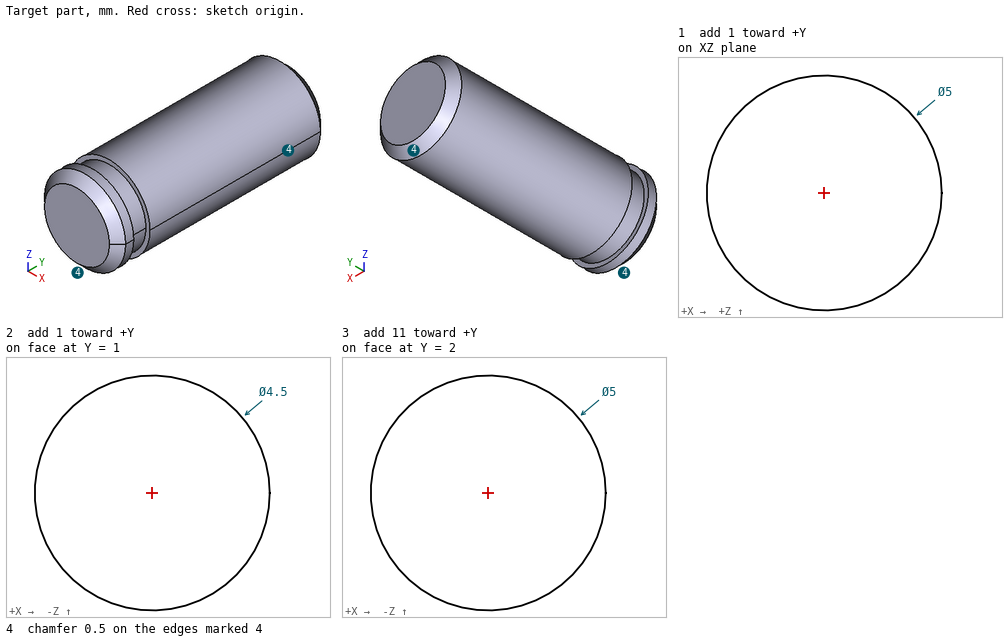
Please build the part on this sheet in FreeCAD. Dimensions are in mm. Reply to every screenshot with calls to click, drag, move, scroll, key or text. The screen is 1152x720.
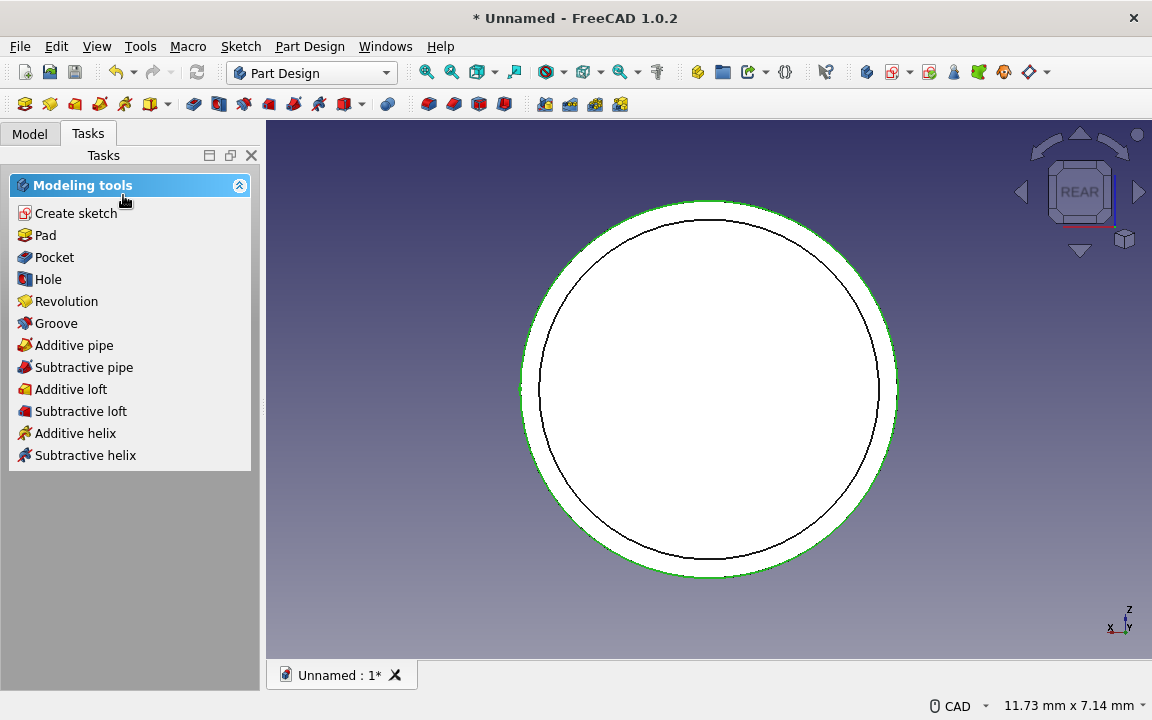
click(25, 104)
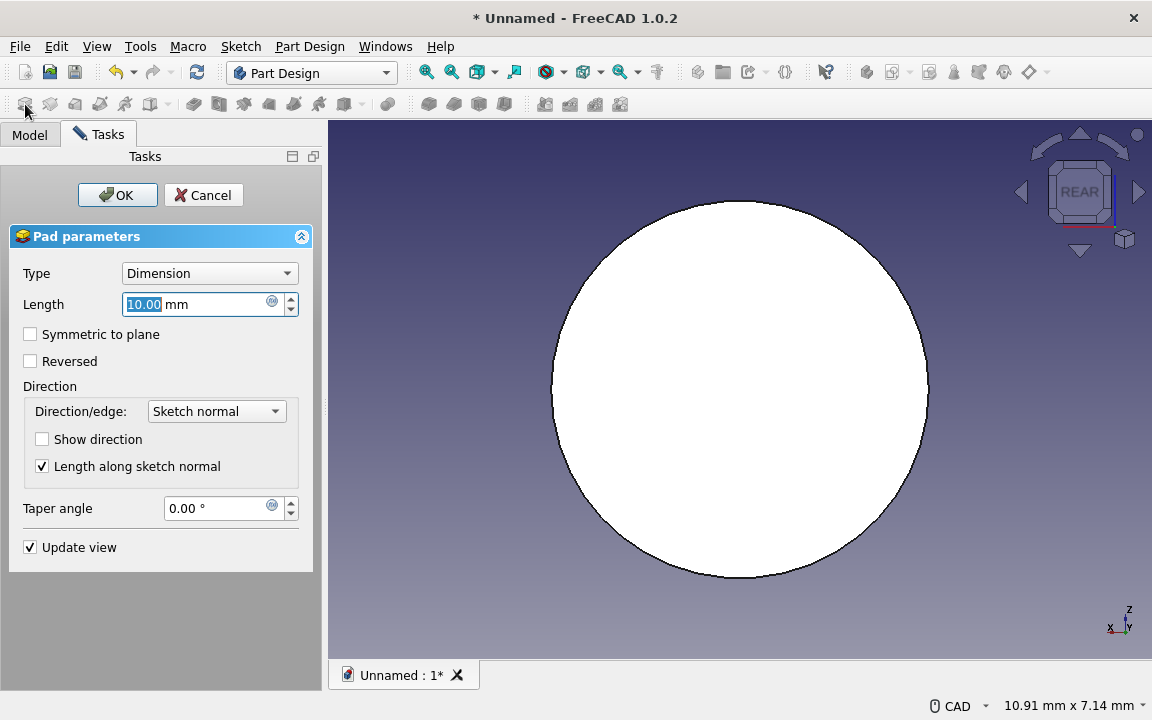
text(11)
key(Tab)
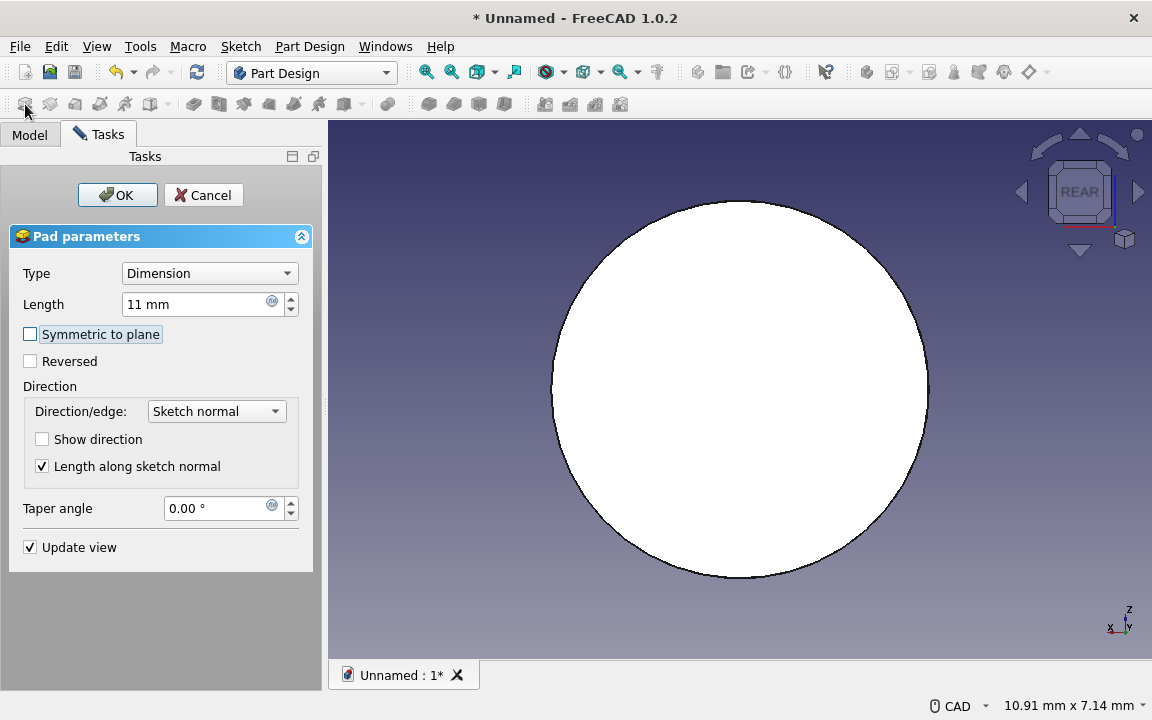
click(118, 195)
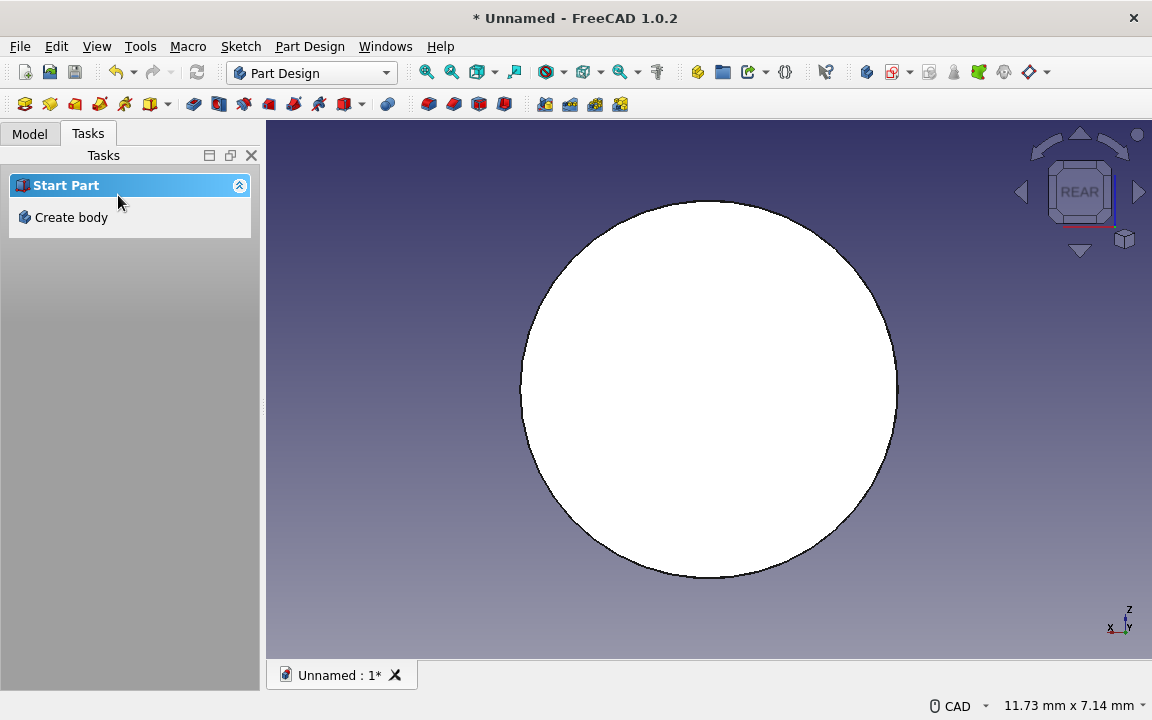
click(898, 389)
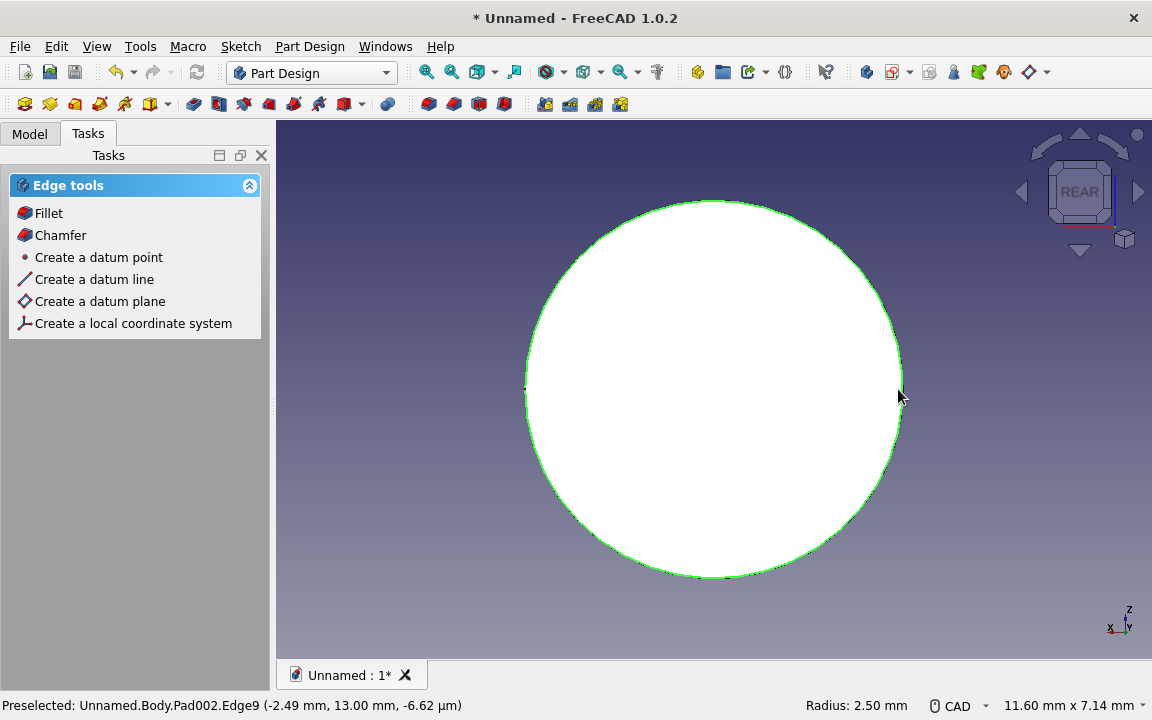
key(0)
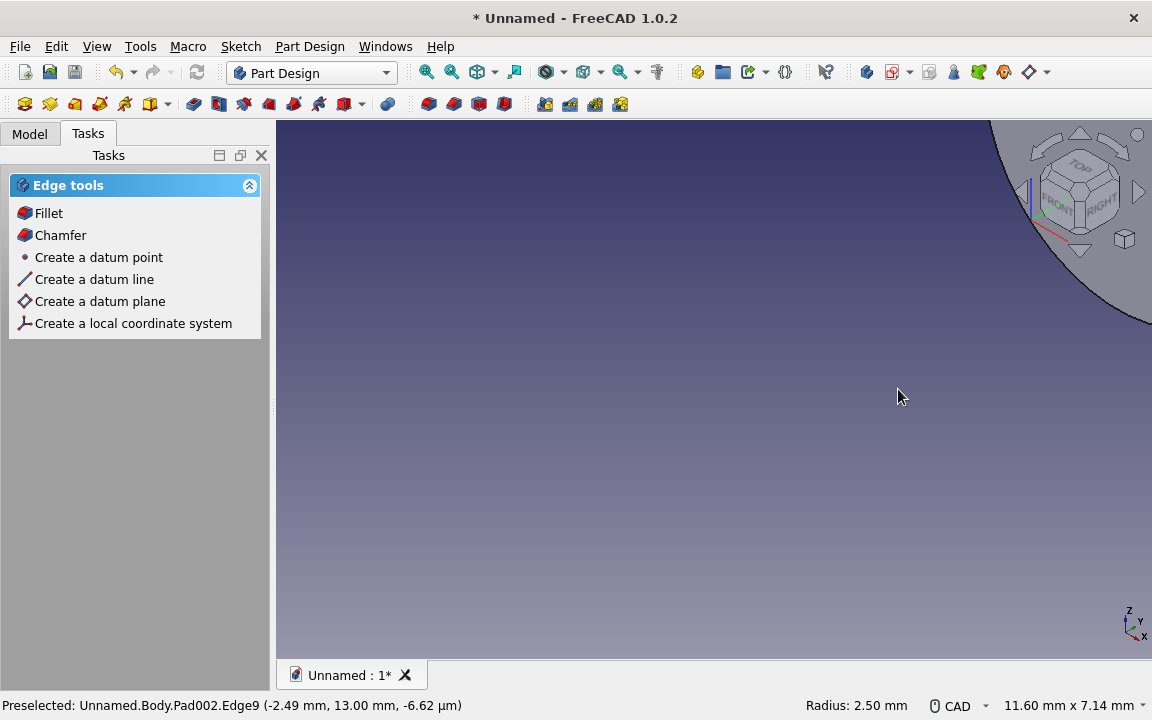
key(v)
key(f)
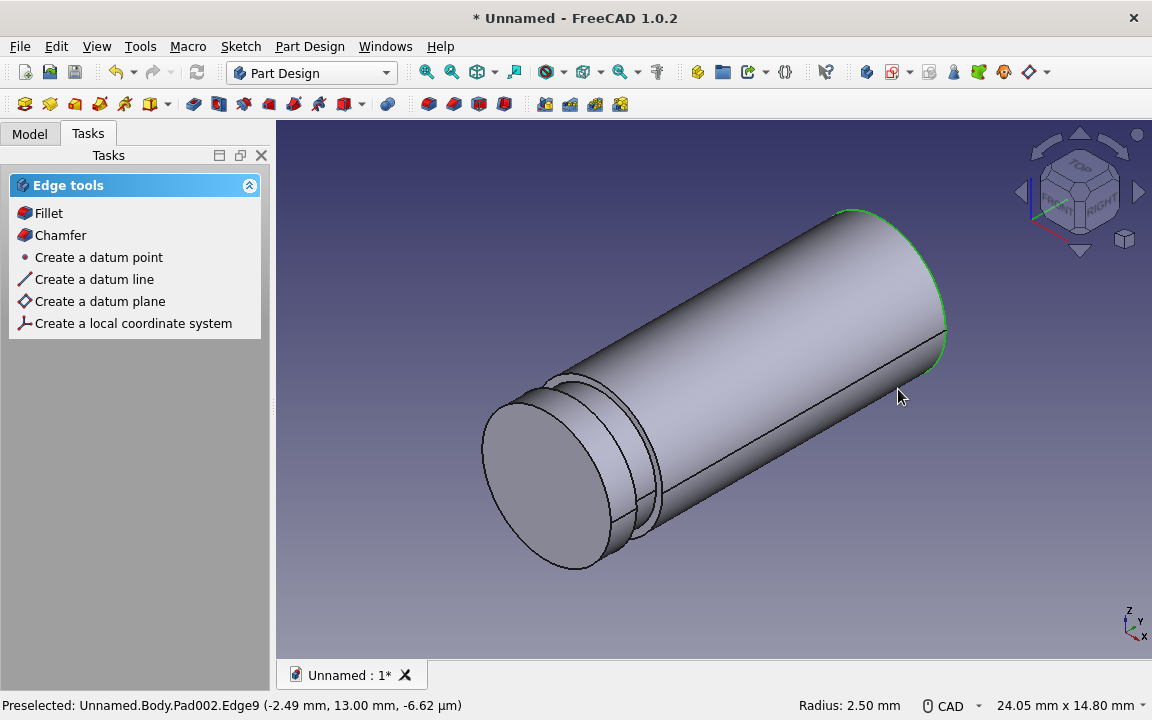
click(527, 403, ctrl)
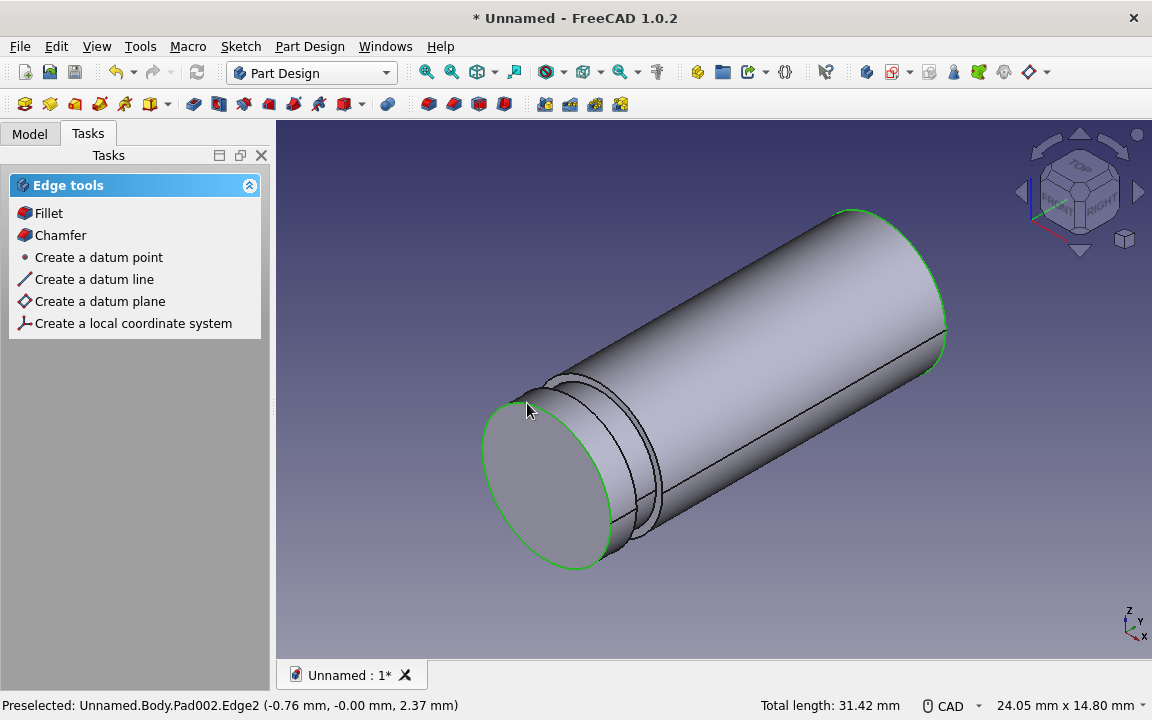
click(454, 104)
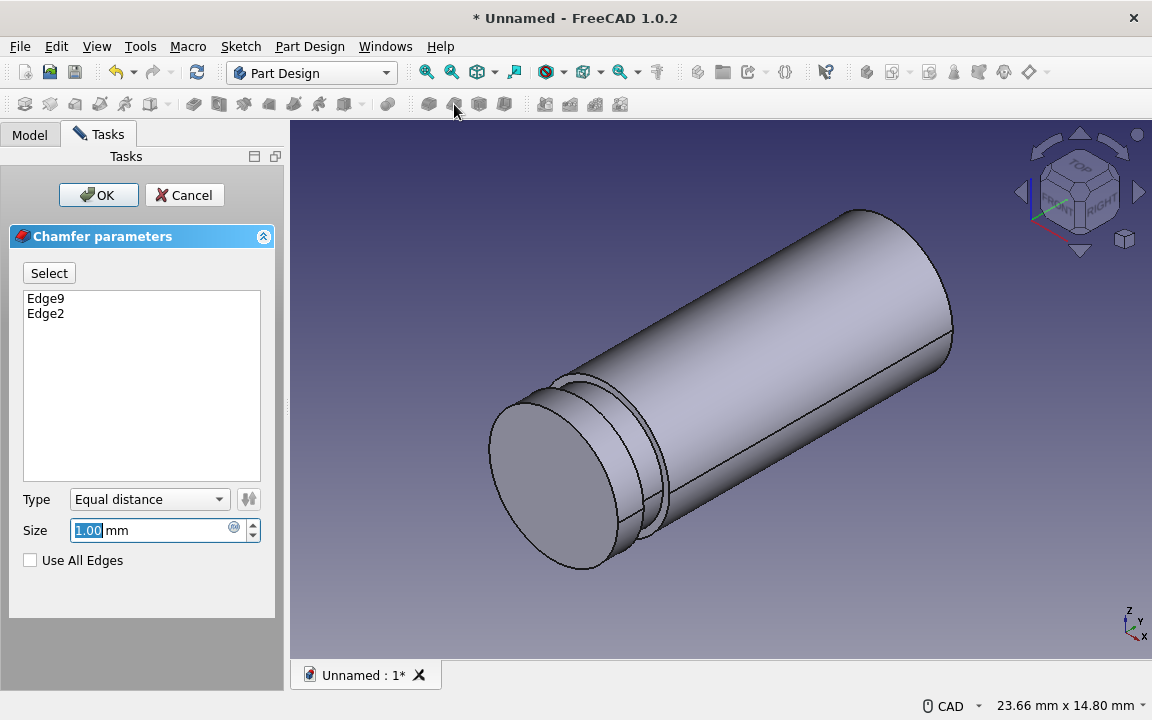
text(0.5)
key(Tab)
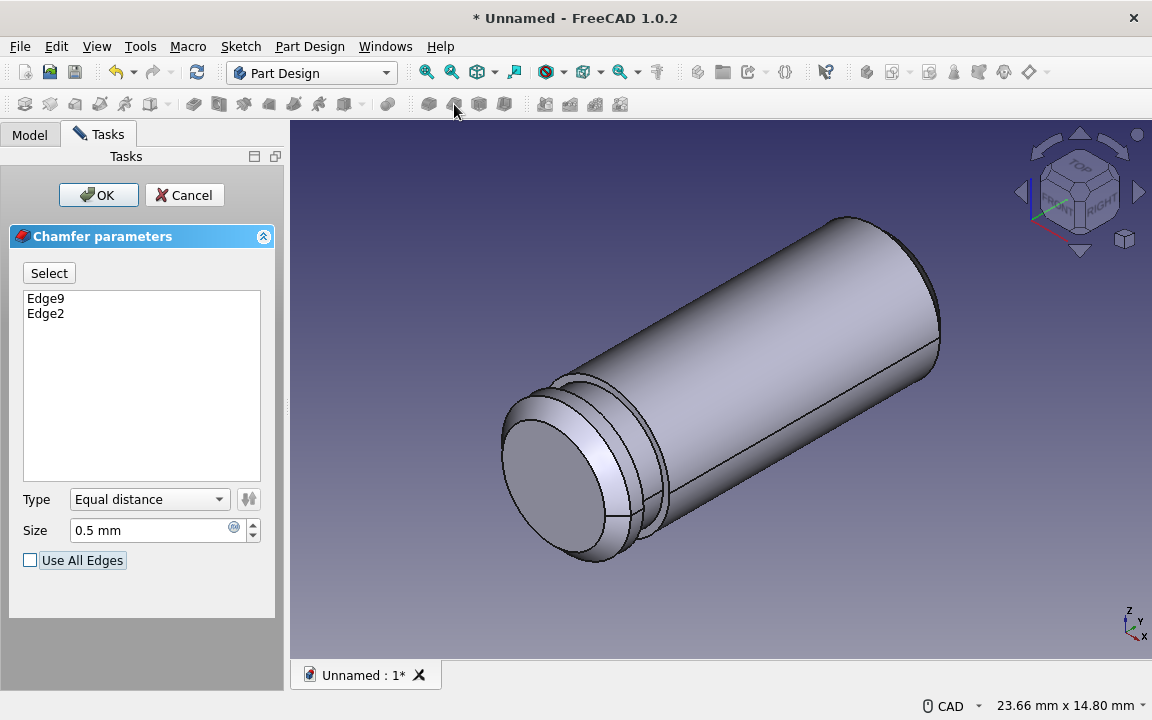
click(99, 195)